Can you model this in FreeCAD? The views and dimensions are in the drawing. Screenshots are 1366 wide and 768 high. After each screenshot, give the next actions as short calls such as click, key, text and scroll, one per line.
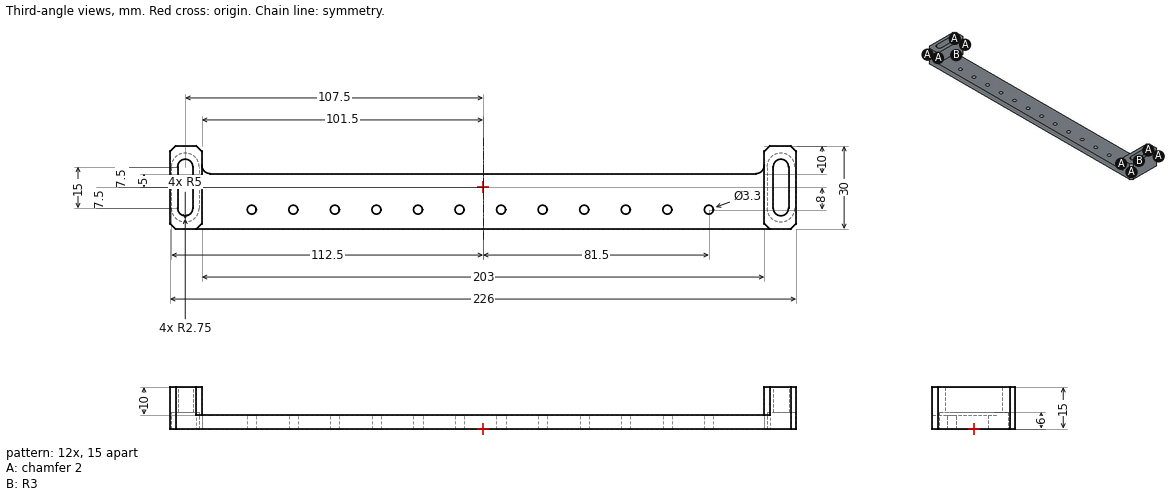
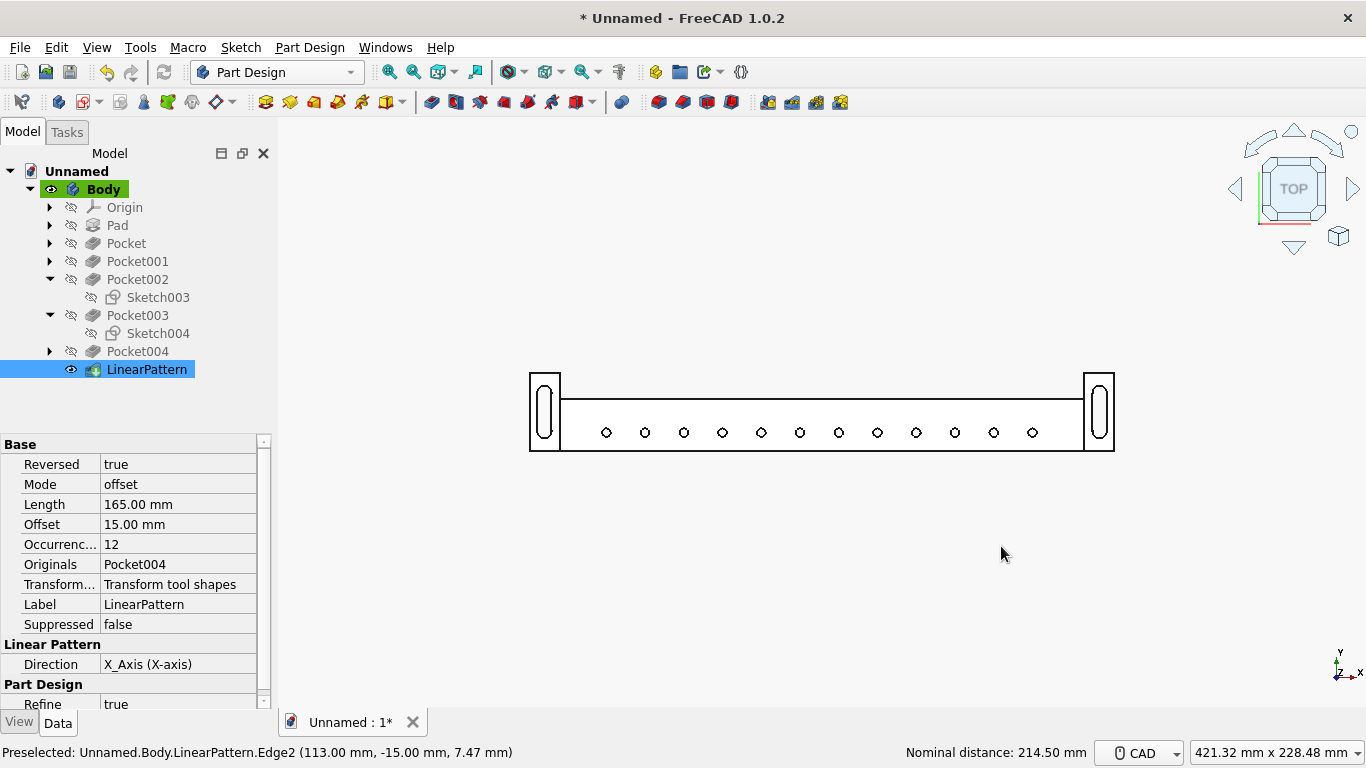
key(1)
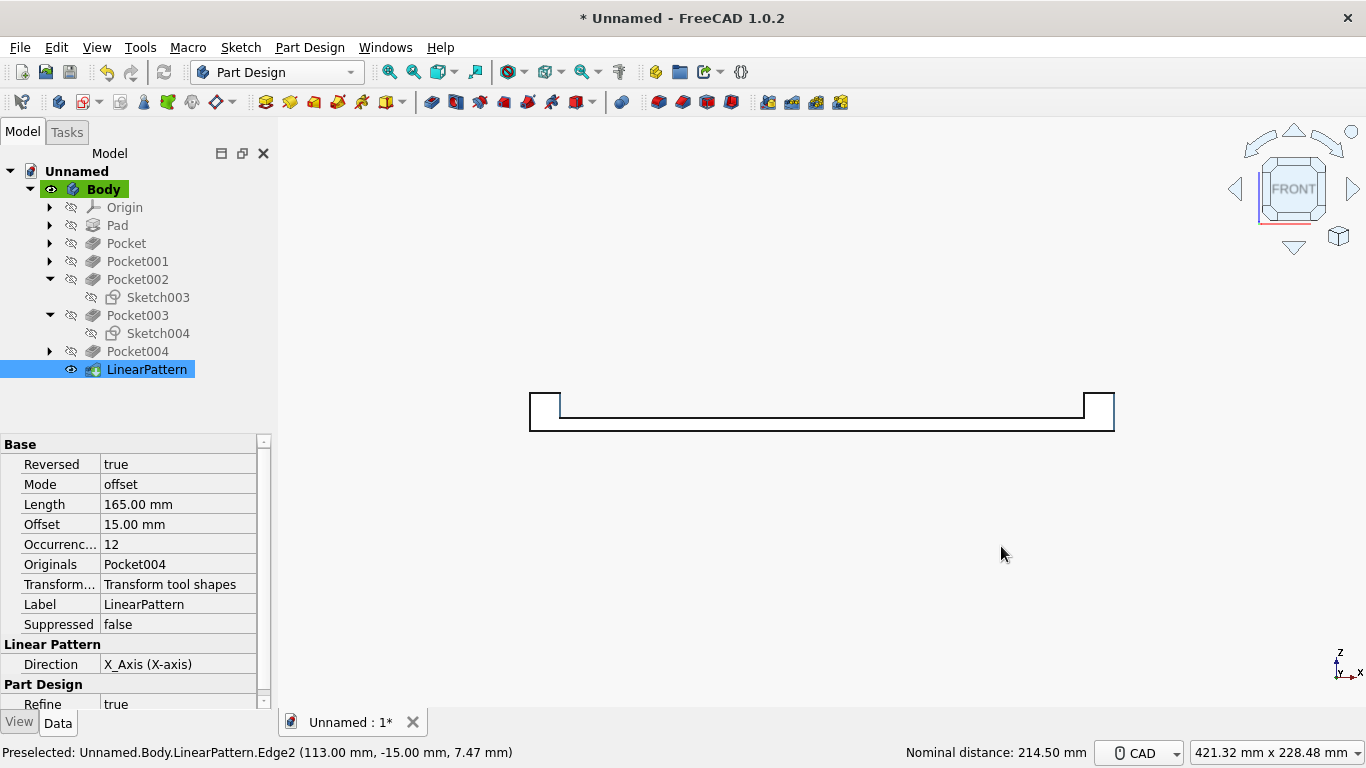
click(1084, 405, ctrl)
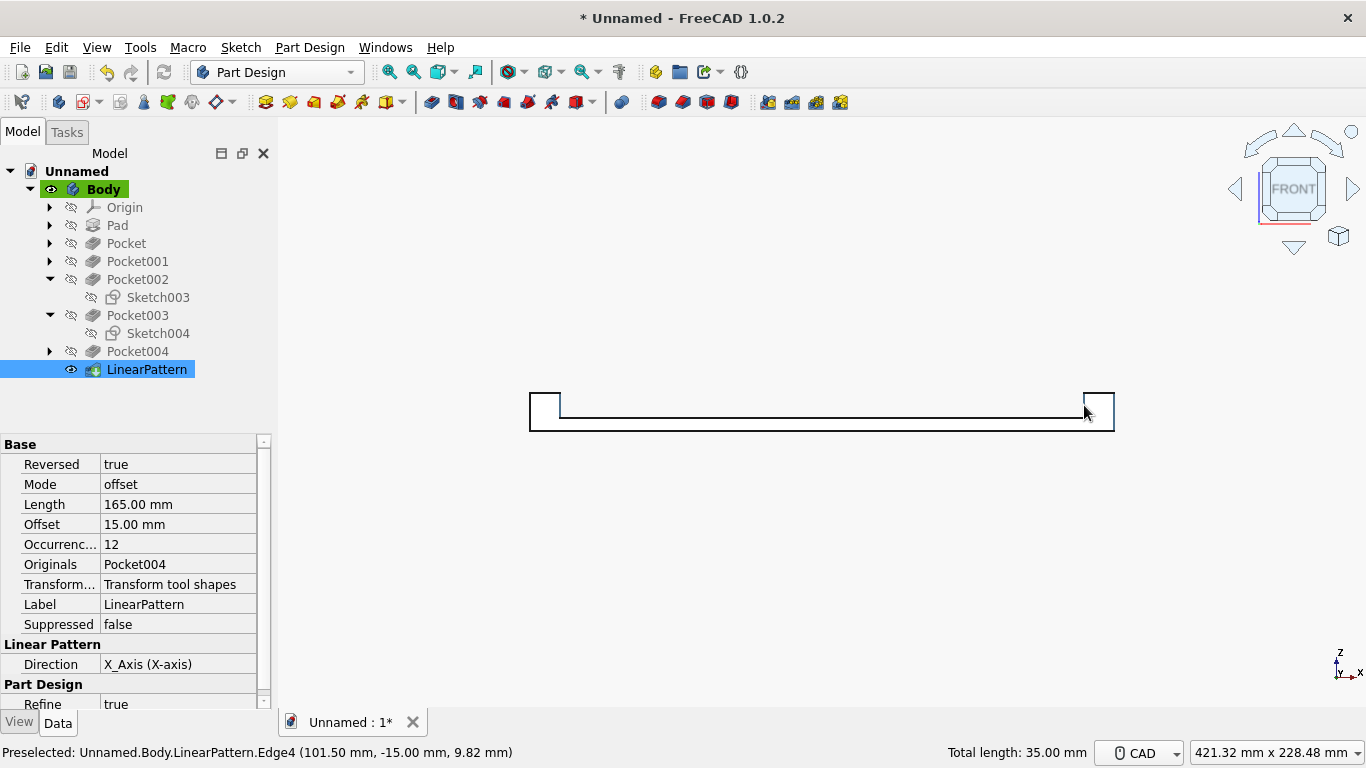
click(530, 411, ctrl)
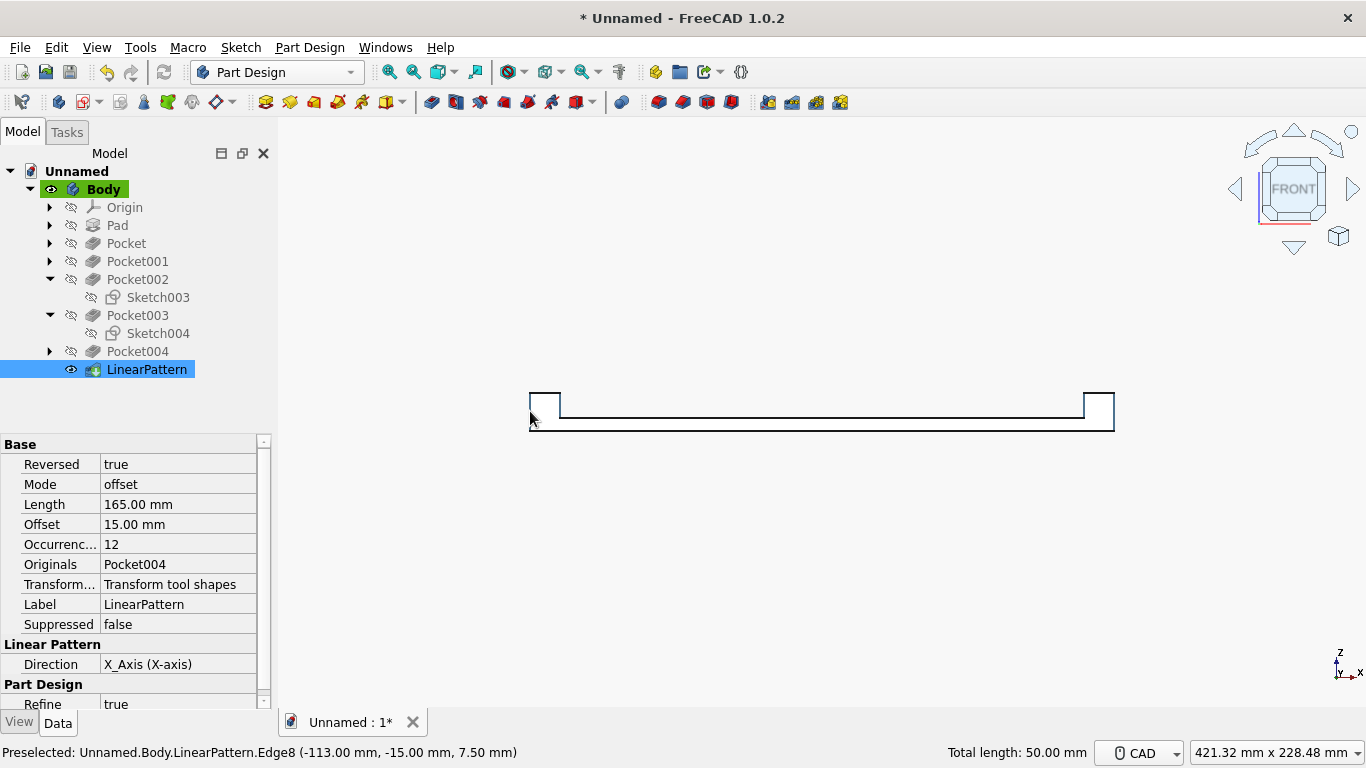
key(3)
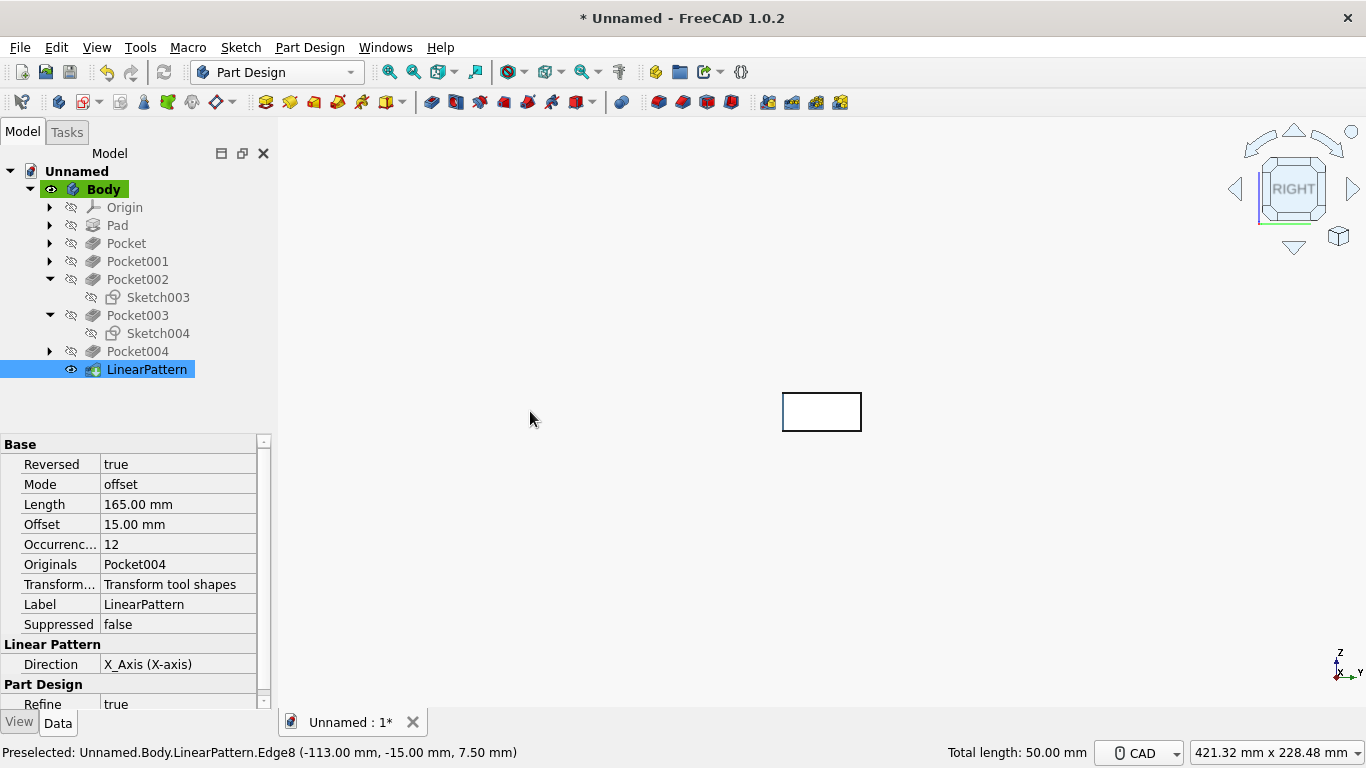
key(v)
key(f)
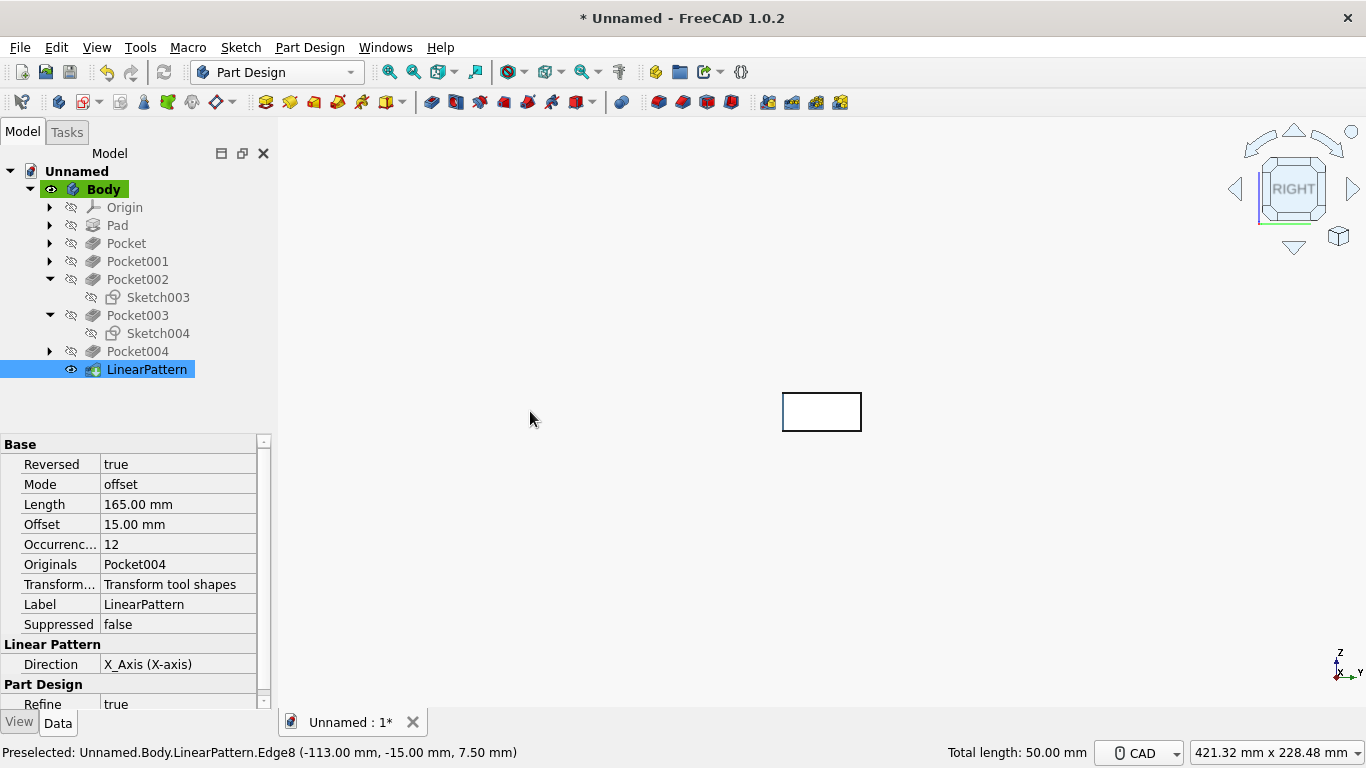
click(861, 411, ctrl)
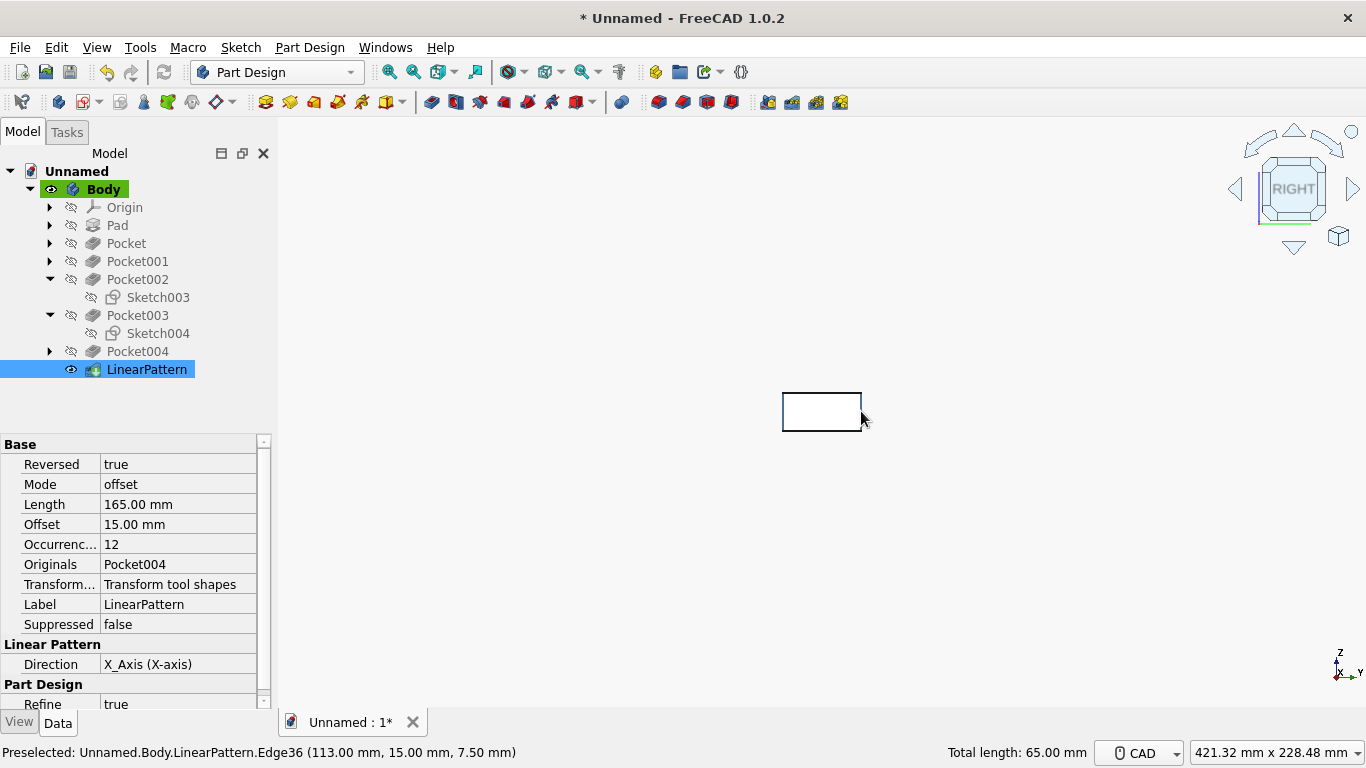
key(5)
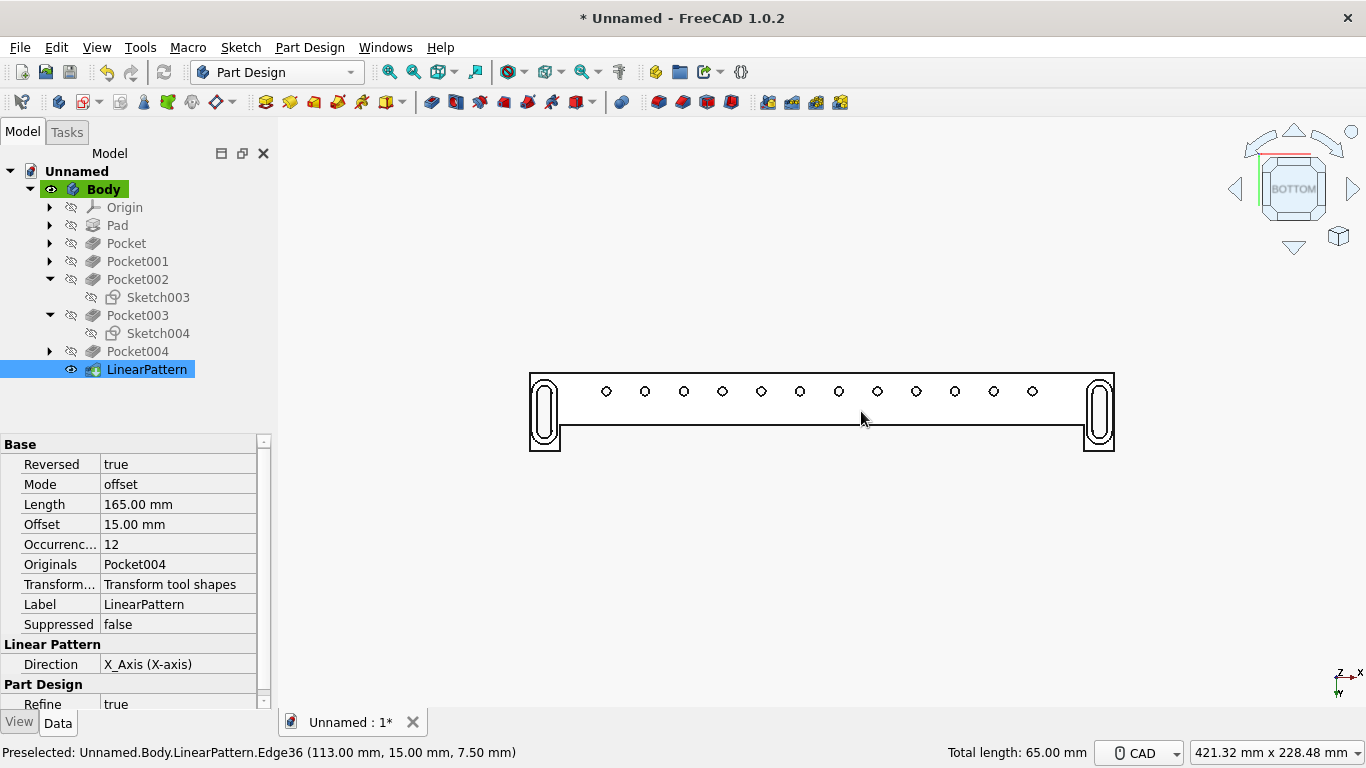
key(4)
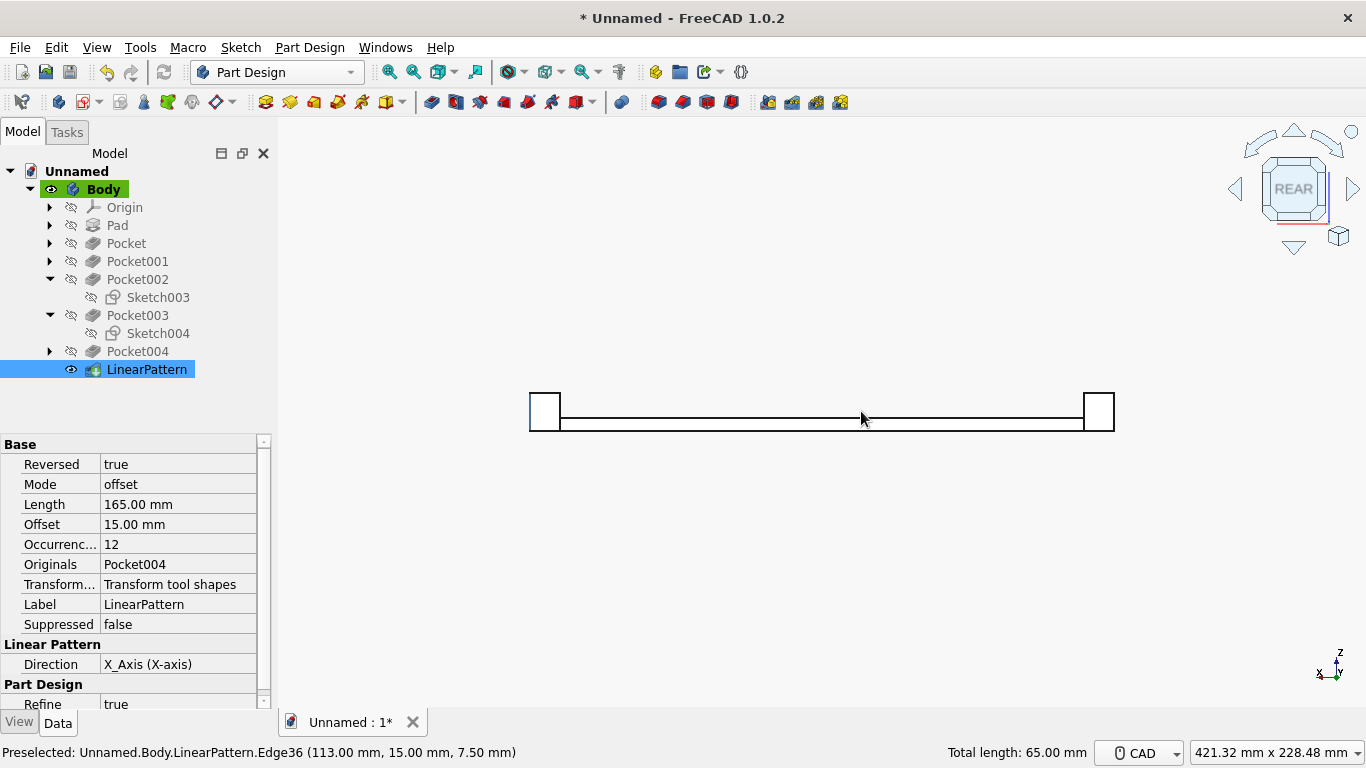
click(560, 411, ctrl)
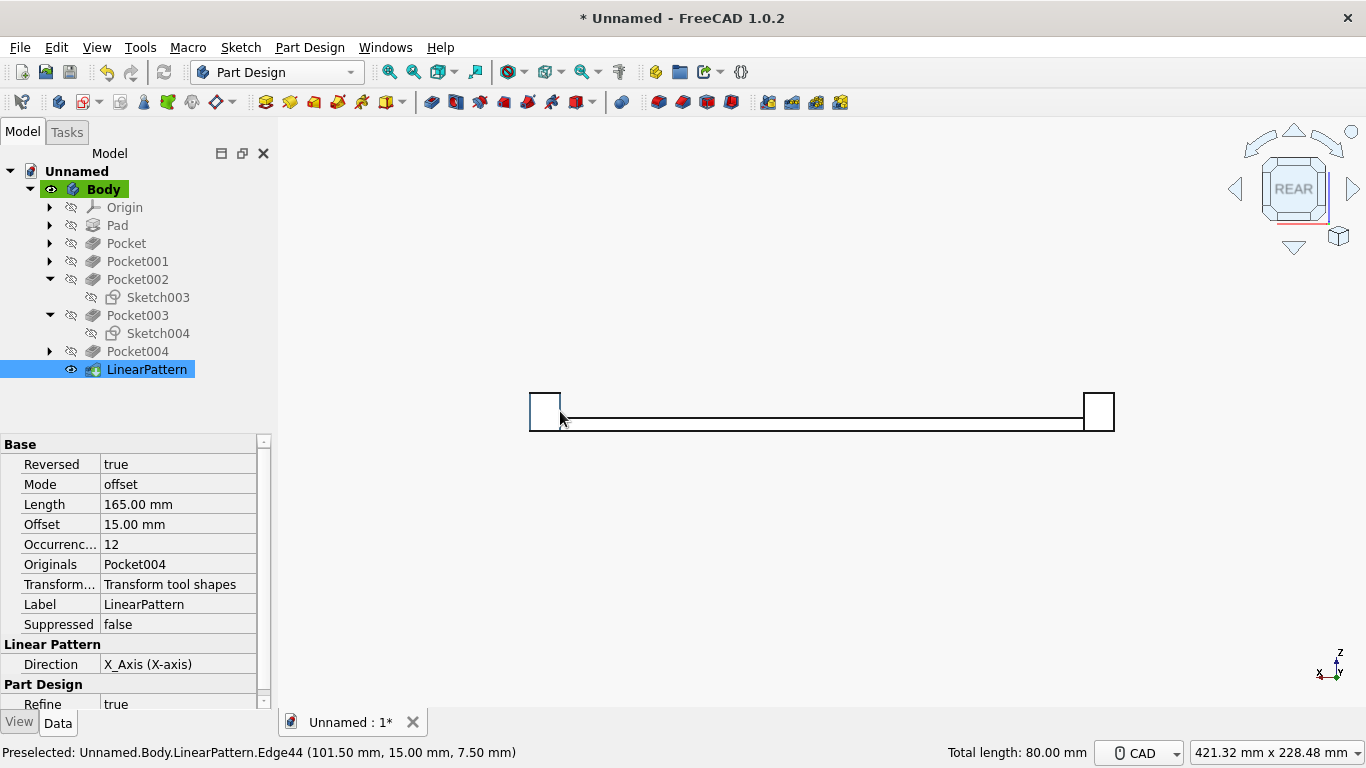
click(1084, 411, ctrl)